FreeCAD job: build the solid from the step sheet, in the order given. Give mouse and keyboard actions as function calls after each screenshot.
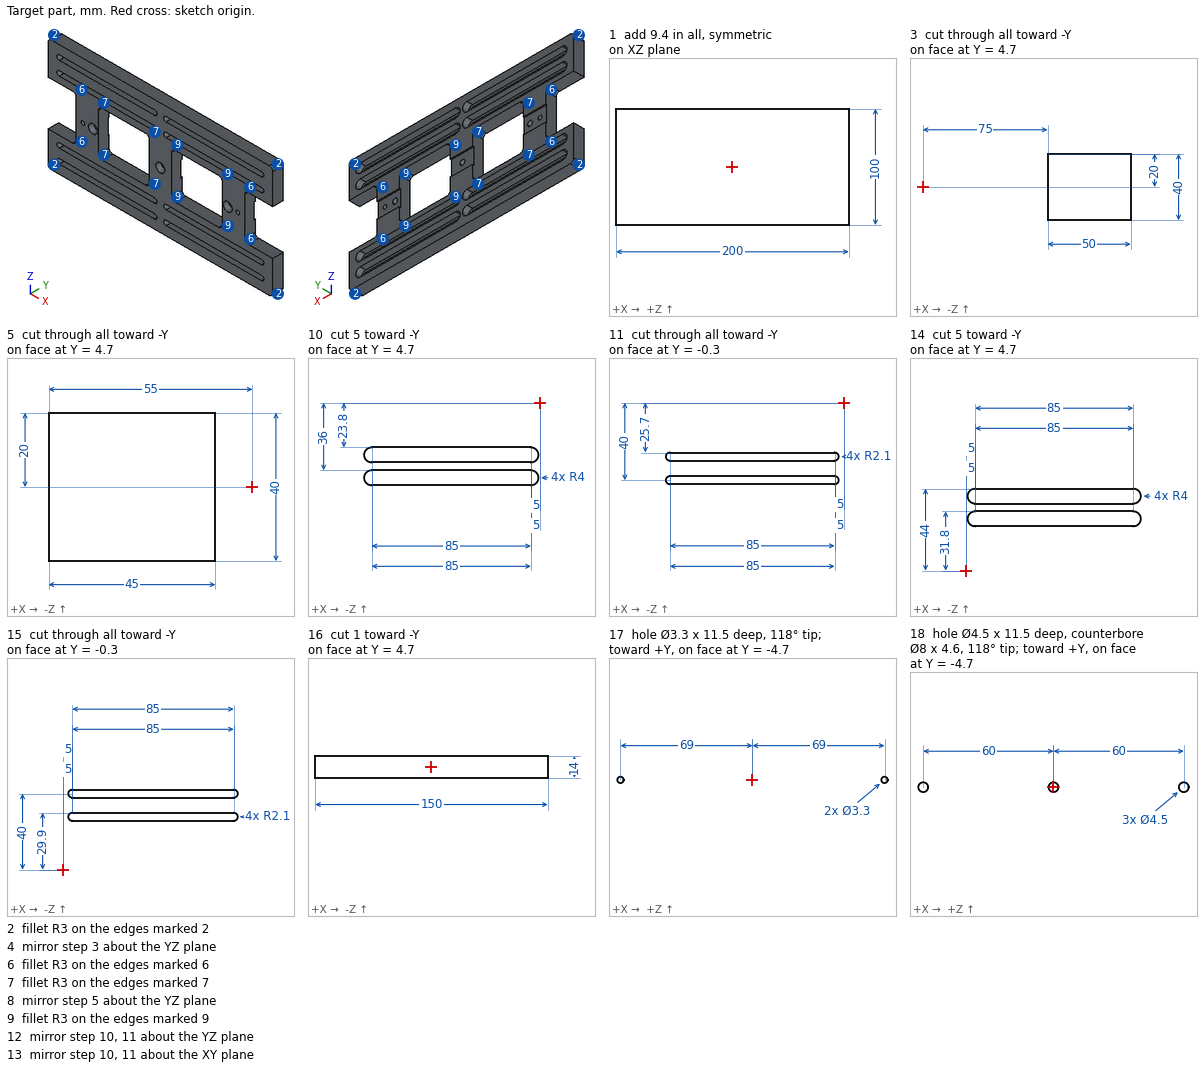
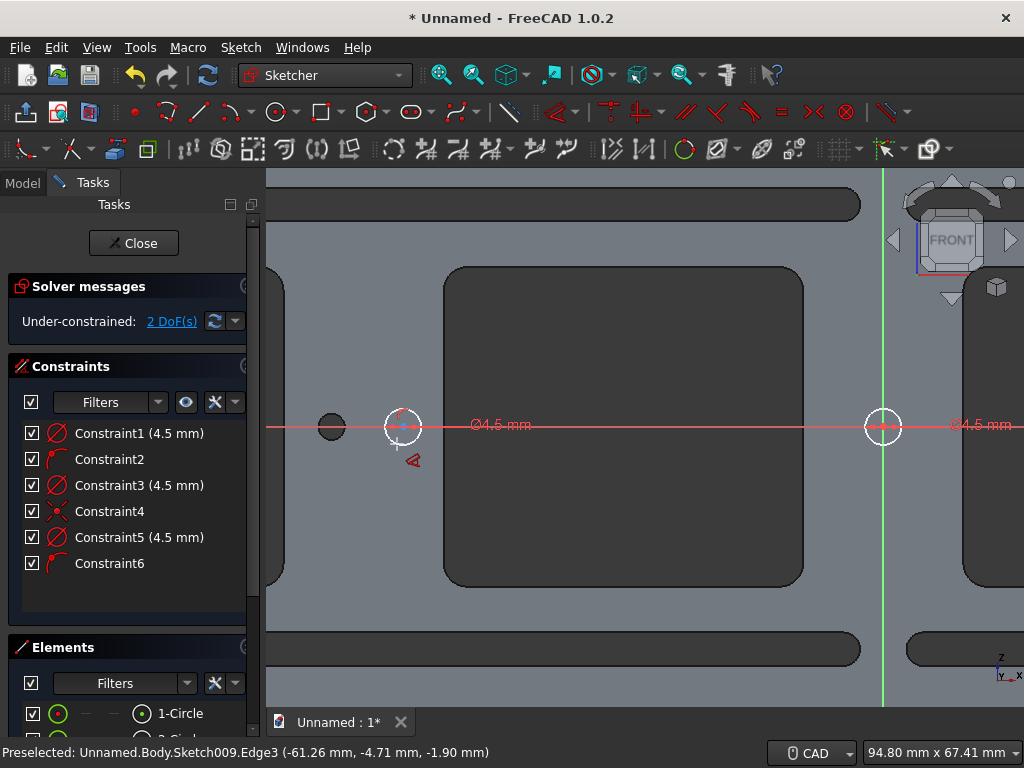
scroll(398, 444, down, 5)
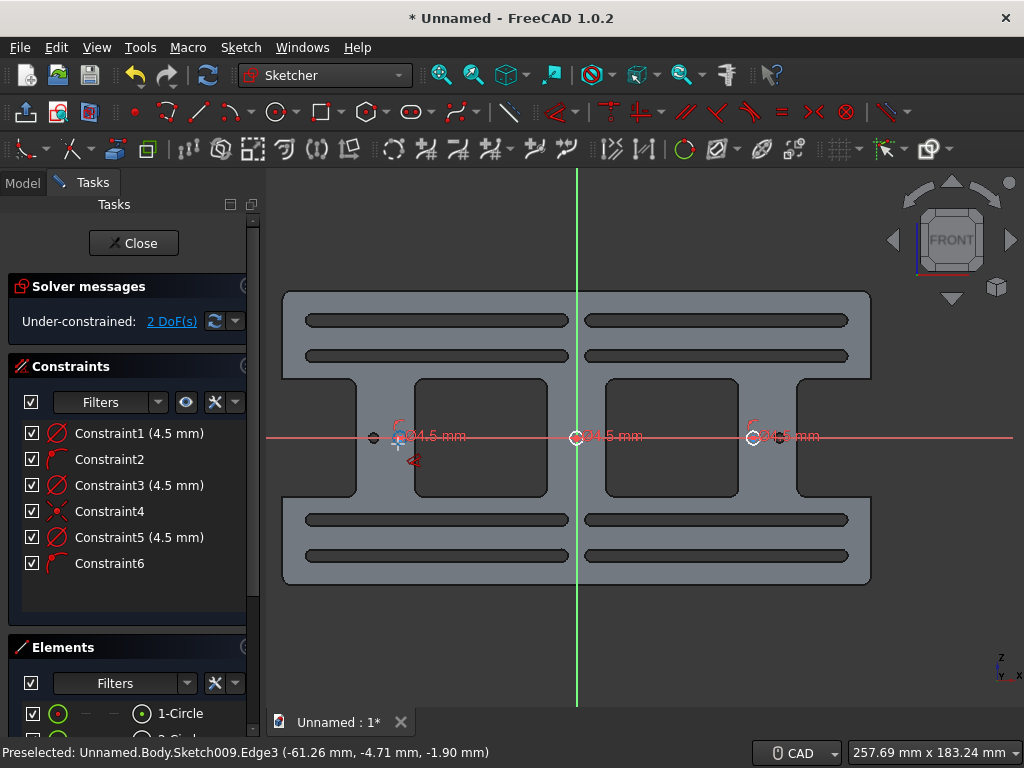
click(753, 438)
click(665, 472)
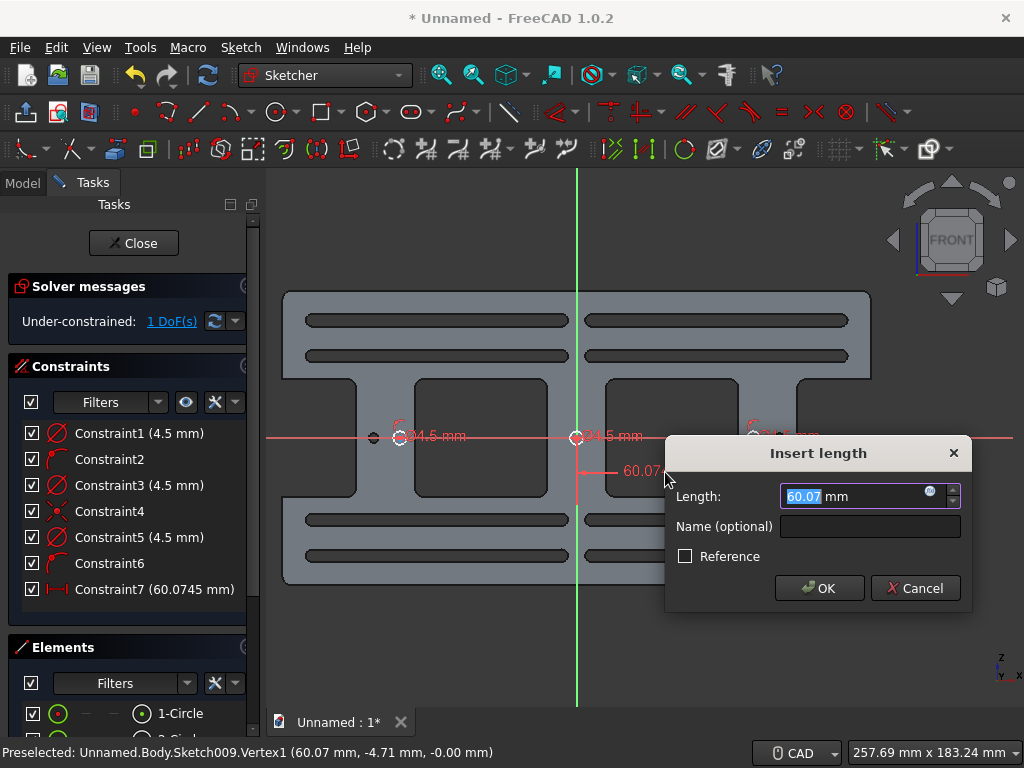
text(60)
key(Return)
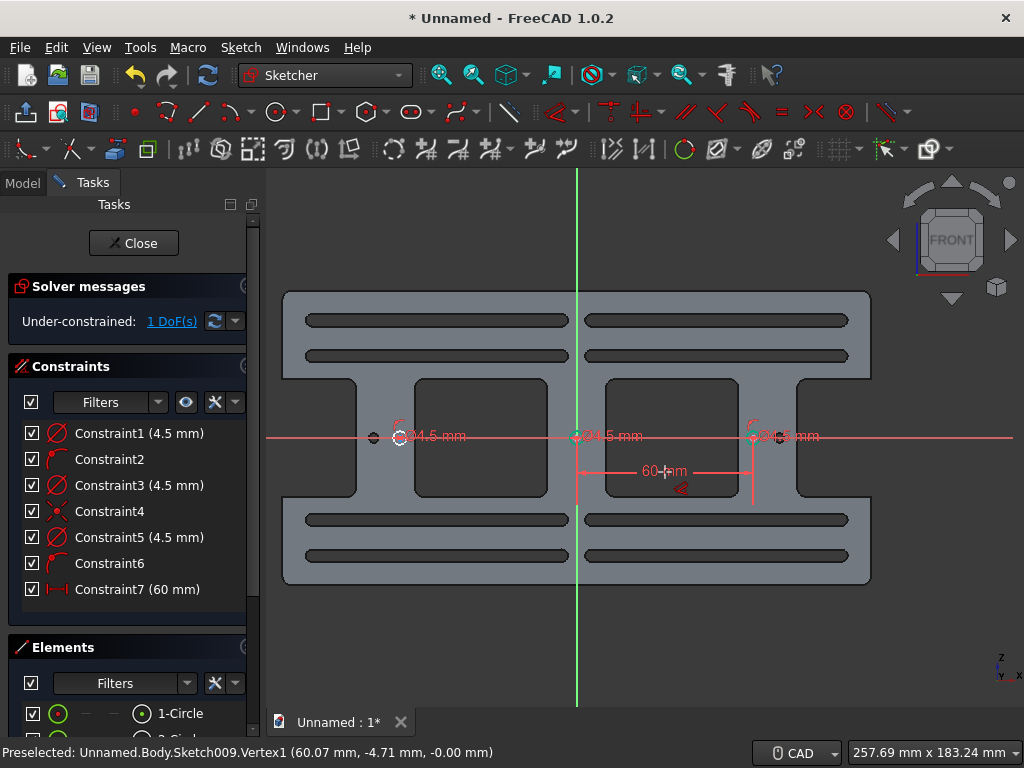
click(400, 438)
click(488, 472)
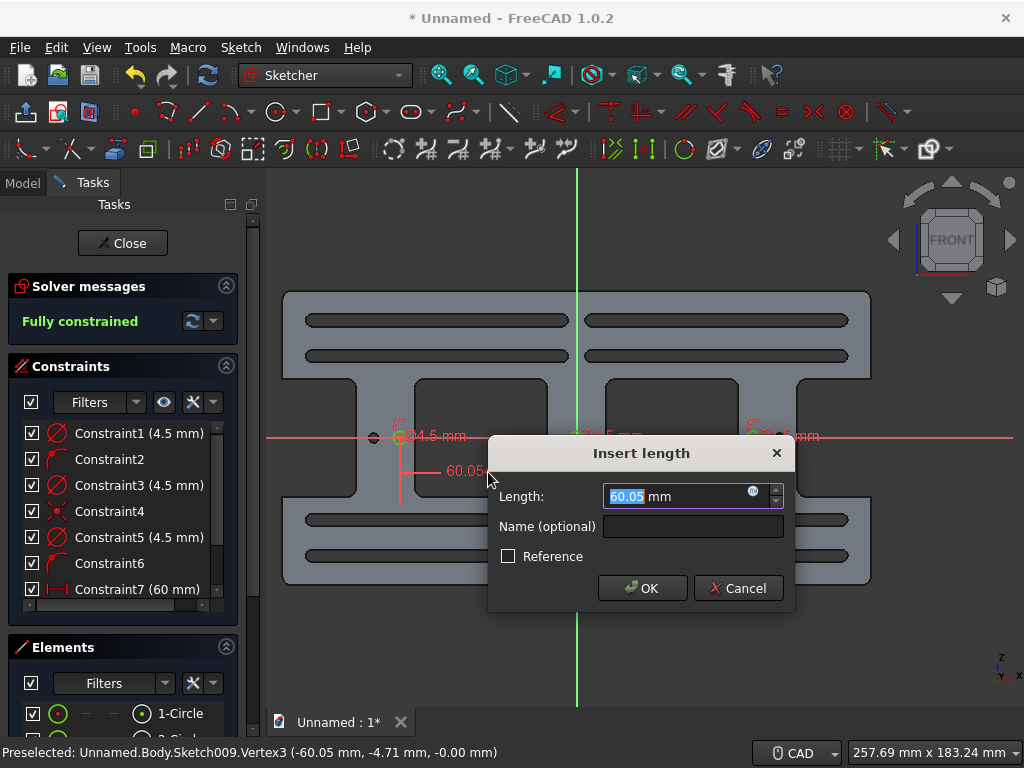
text(60)
key(Return)
key(Escape)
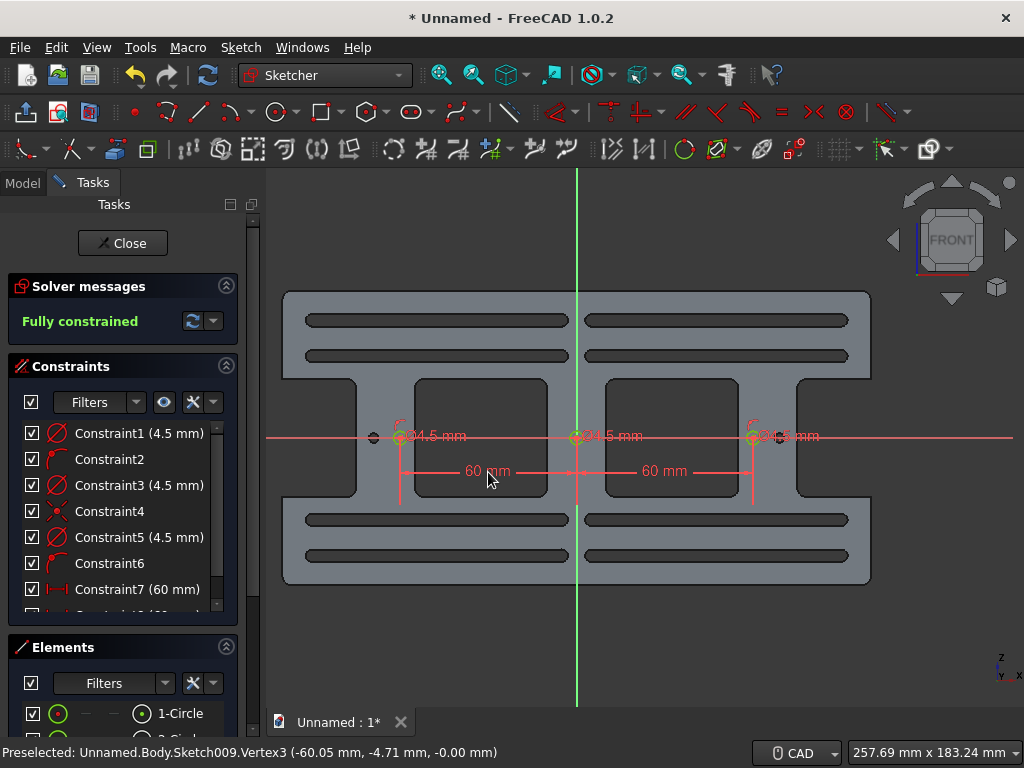
click(123, 243)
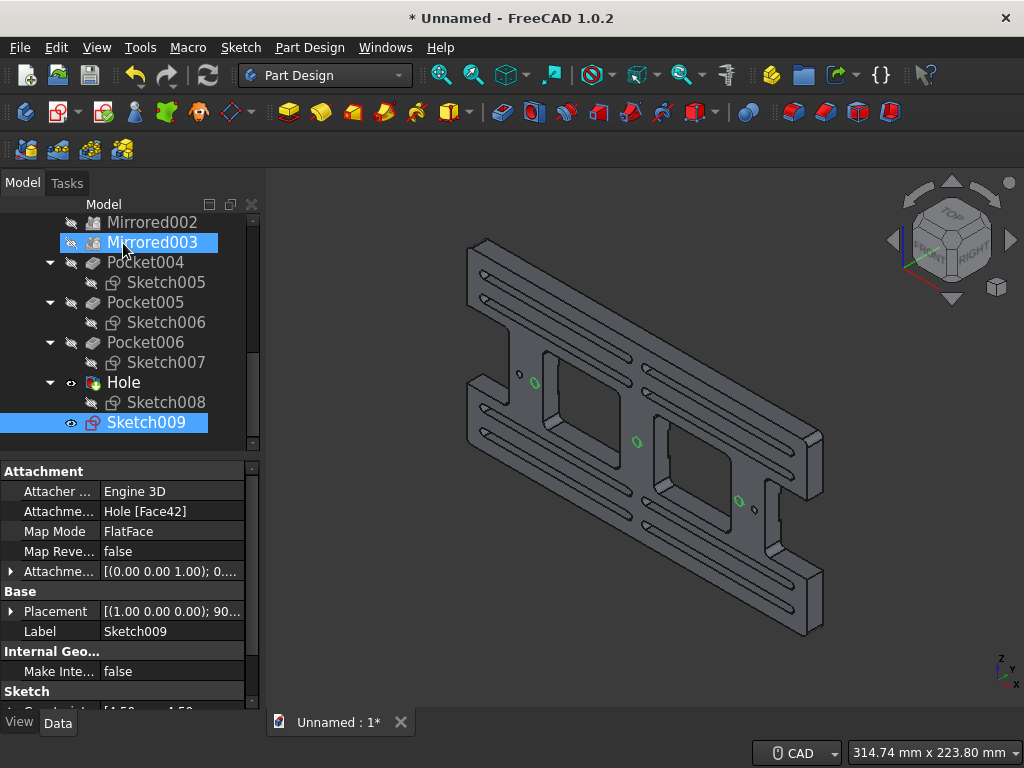
click(536, 112)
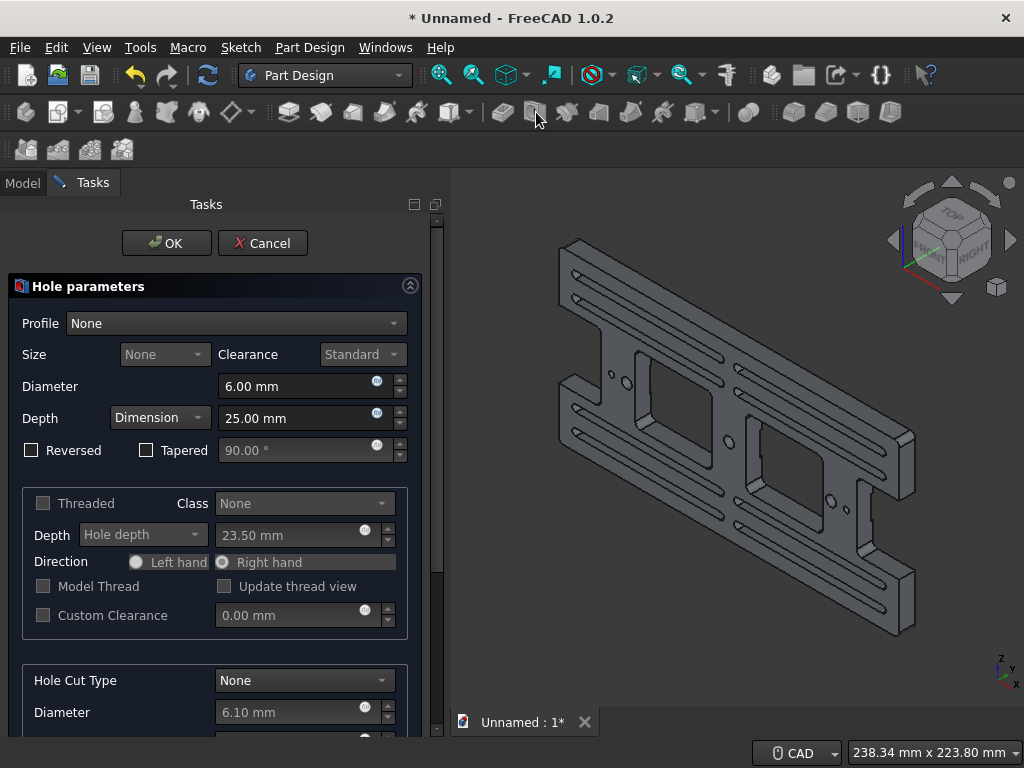
triple_click(305, 386)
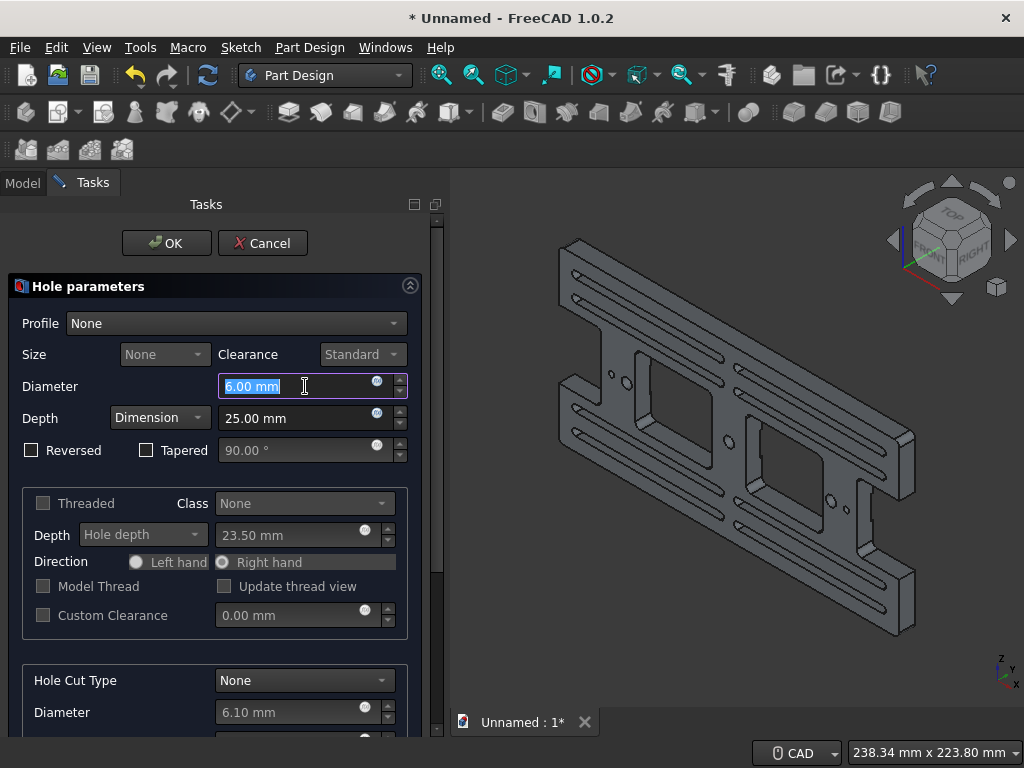
text(4.5)
key(Tab)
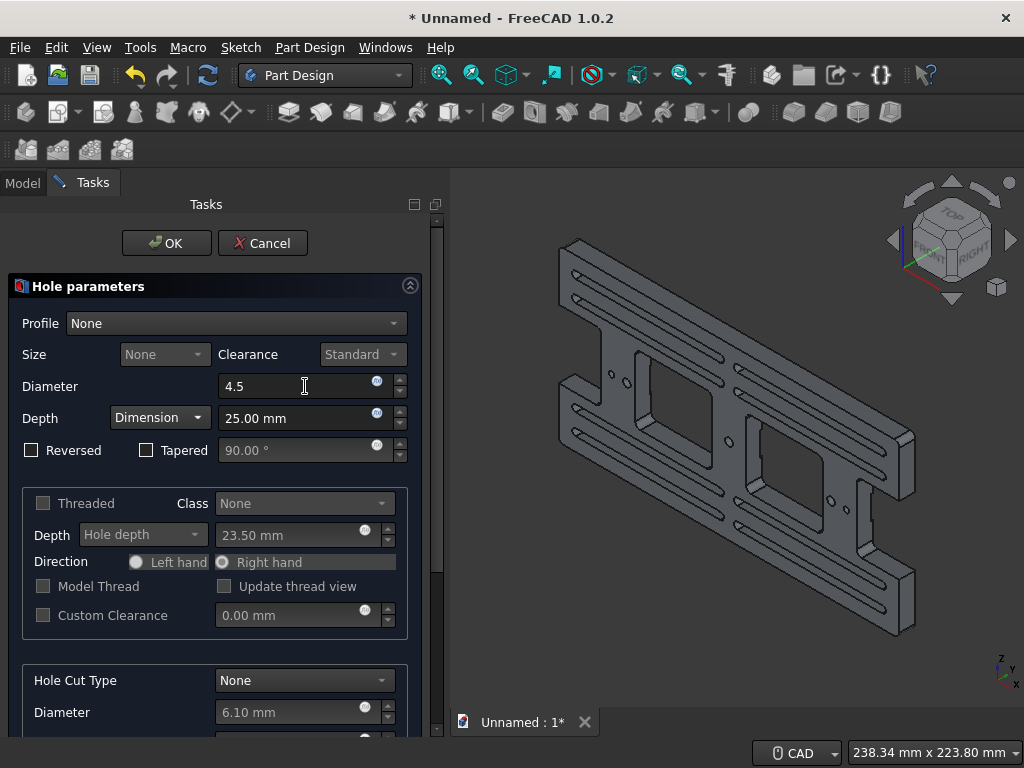
triple_click(305, 418)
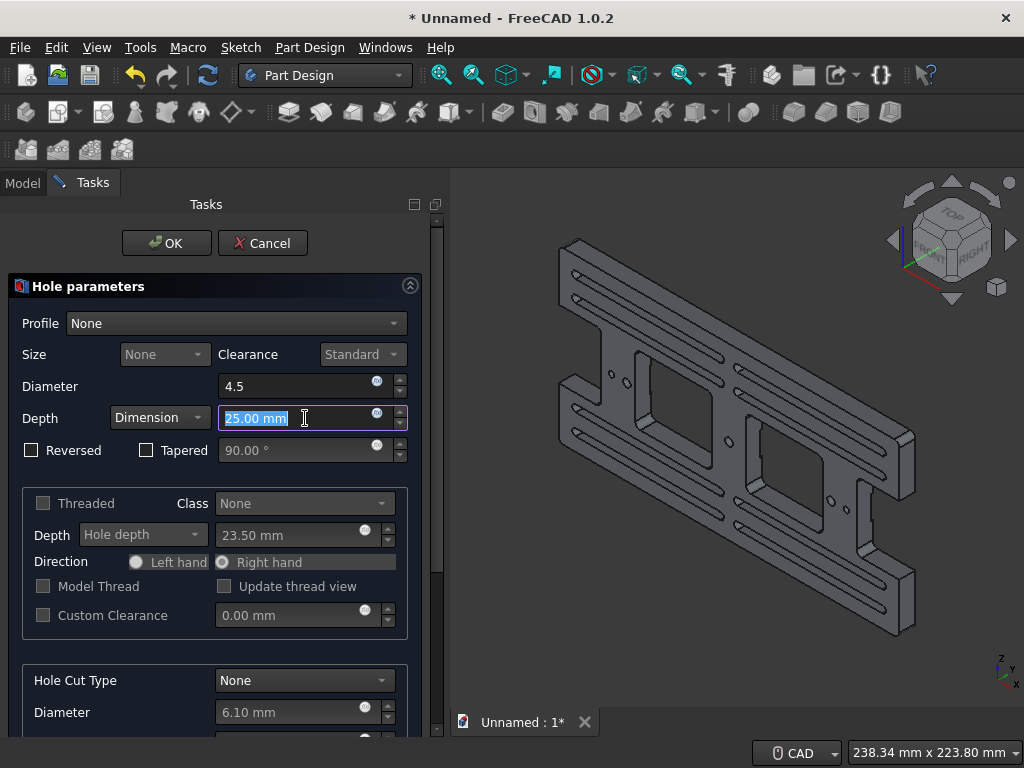
text(11.5)
key(Tab)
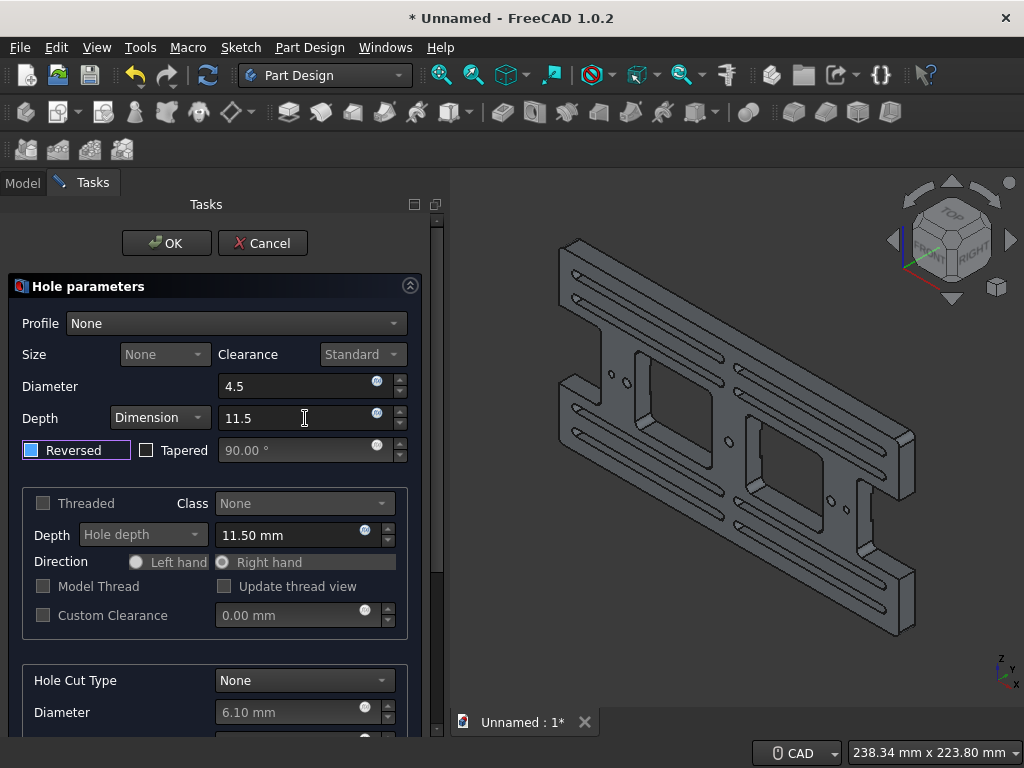
click(306, 680)